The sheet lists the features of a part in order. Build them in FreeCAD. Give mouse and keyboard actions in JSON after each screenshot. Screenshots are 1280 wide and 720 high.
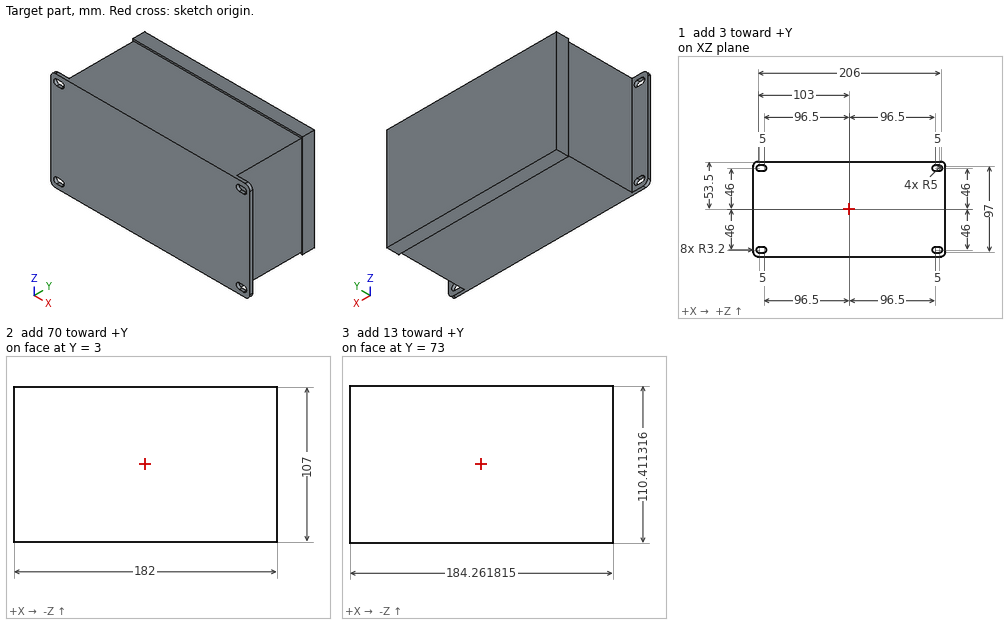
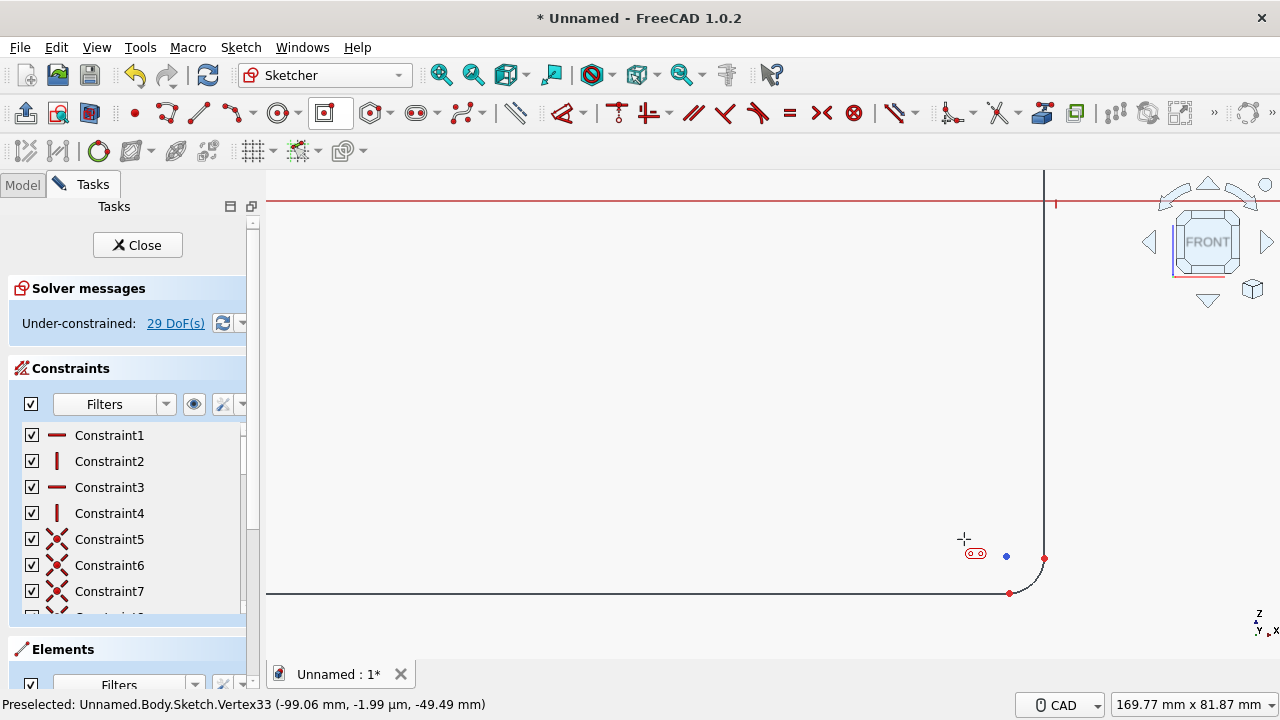
{"action": "left_click", "coordinate": [962, 537]}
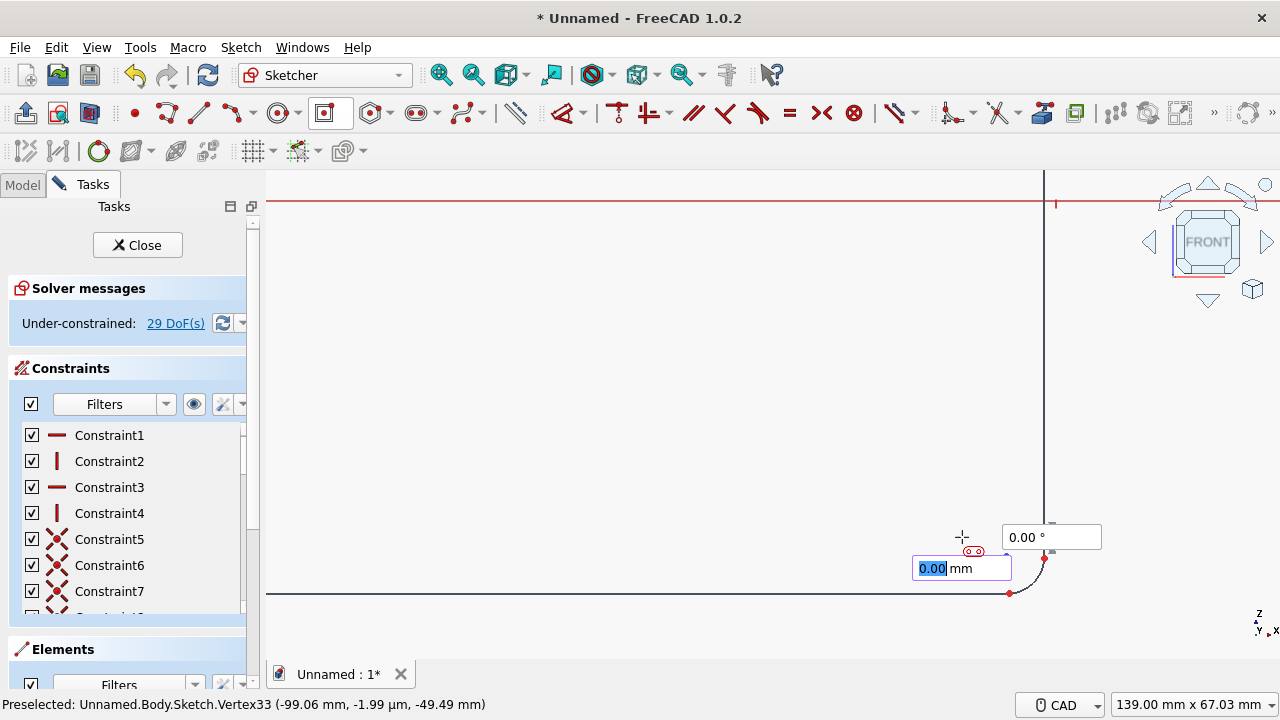
{"action": "left_click", "coordinate": [998, 537]}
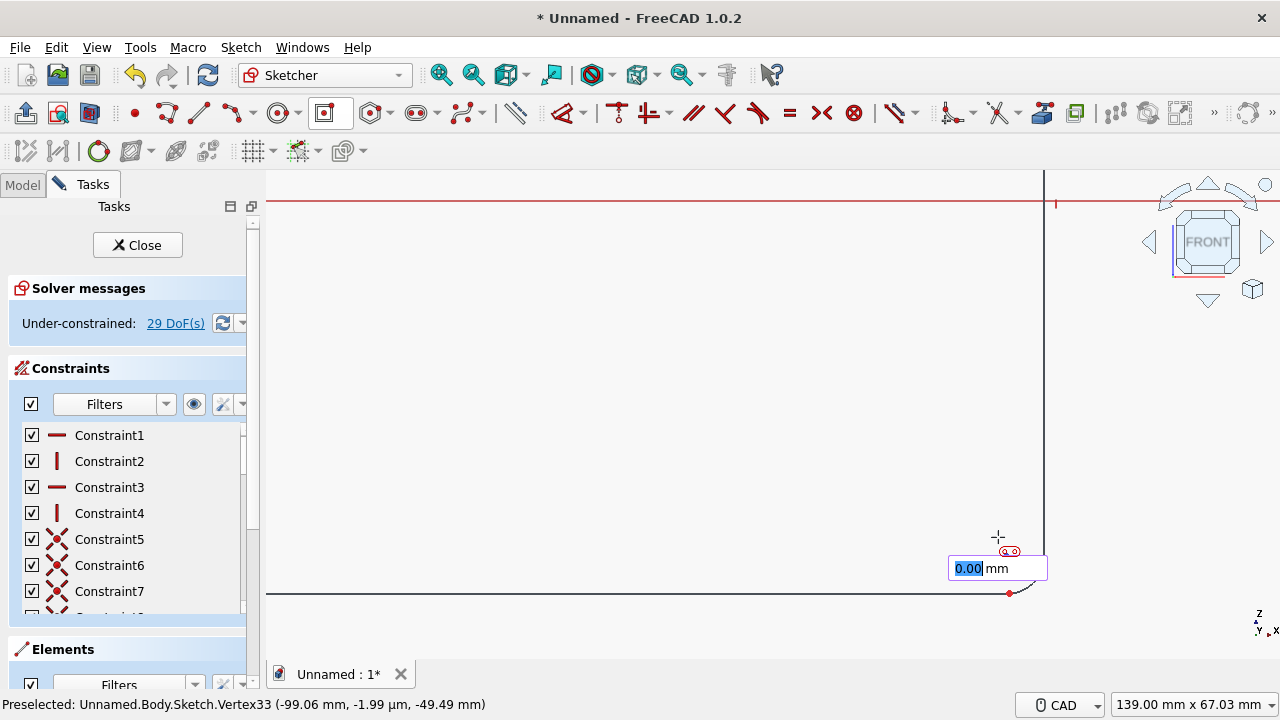
{"action": "left_click", "coordinate": [980, 560]}
{"action": "key", "text": "Escape"}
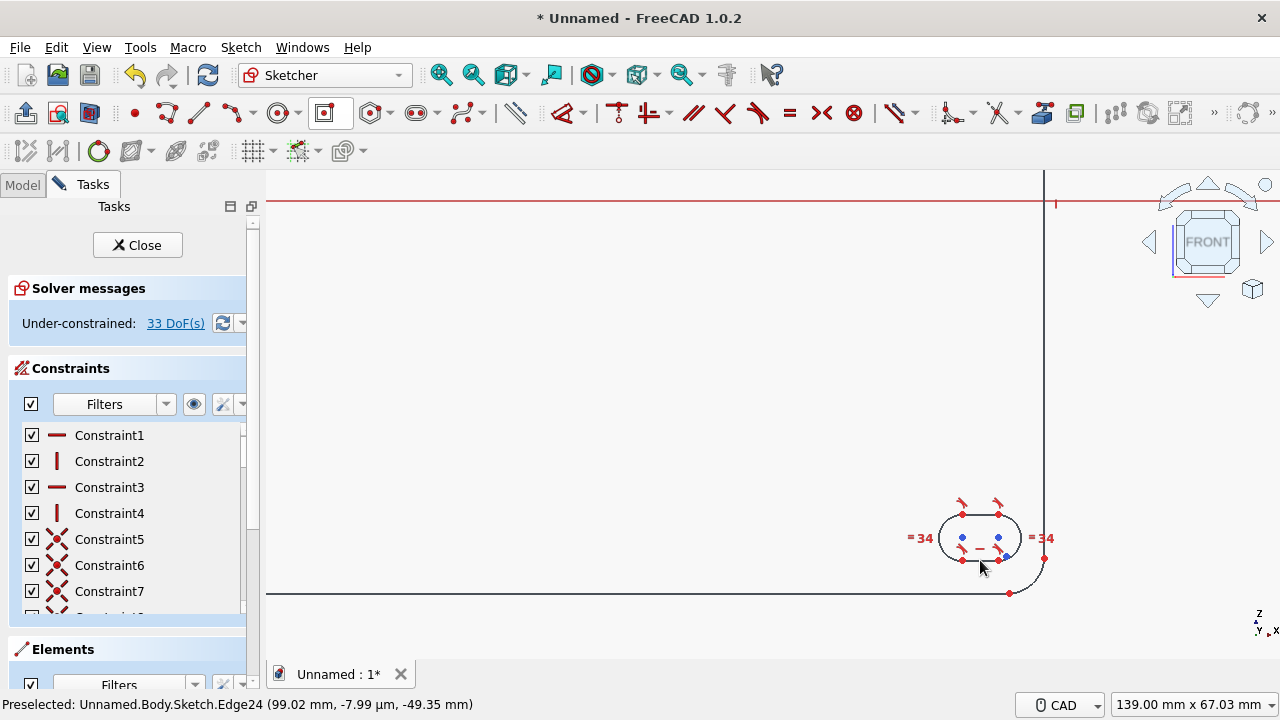
{"action": "scroll", "coordinate": [965, 539], "scroll_direction": "down", "scroll_amount": 5}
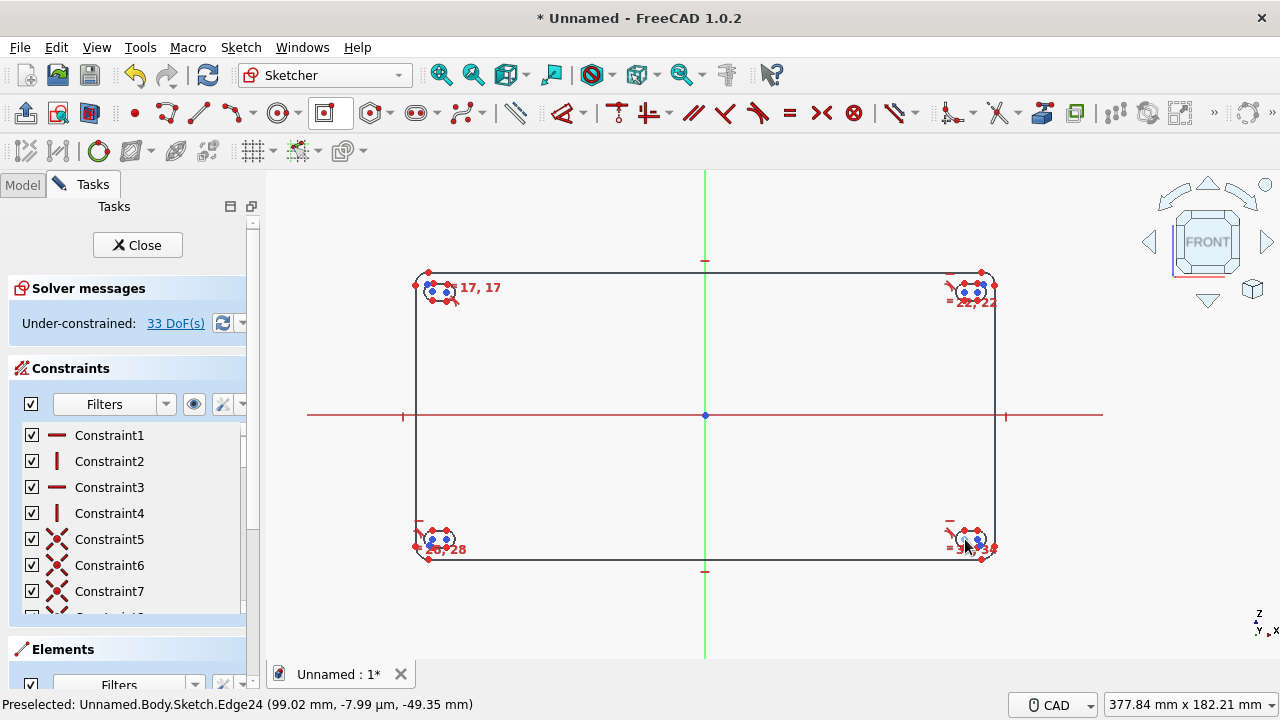
{"action": "left_click", "coordinate": [595, 273]}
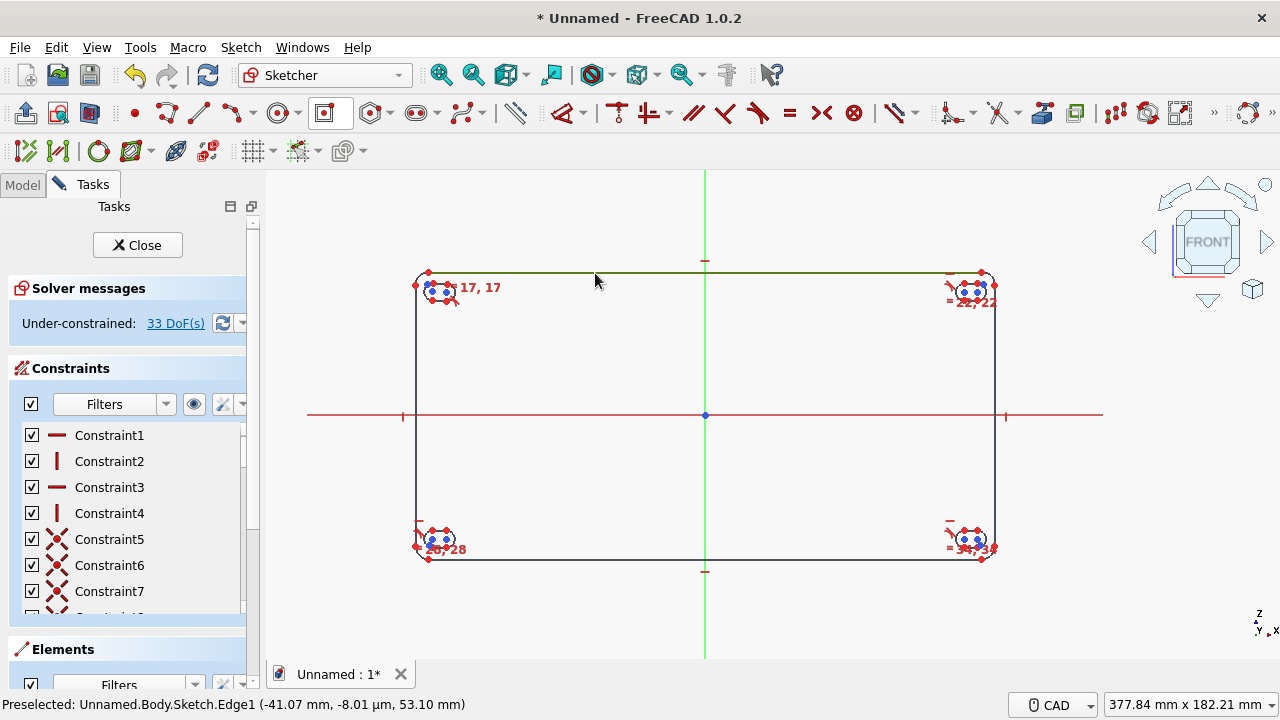
{"action": "scroll", "coordinate": [991, 276], "scroll_direction": "up", "scroll_amount": 2}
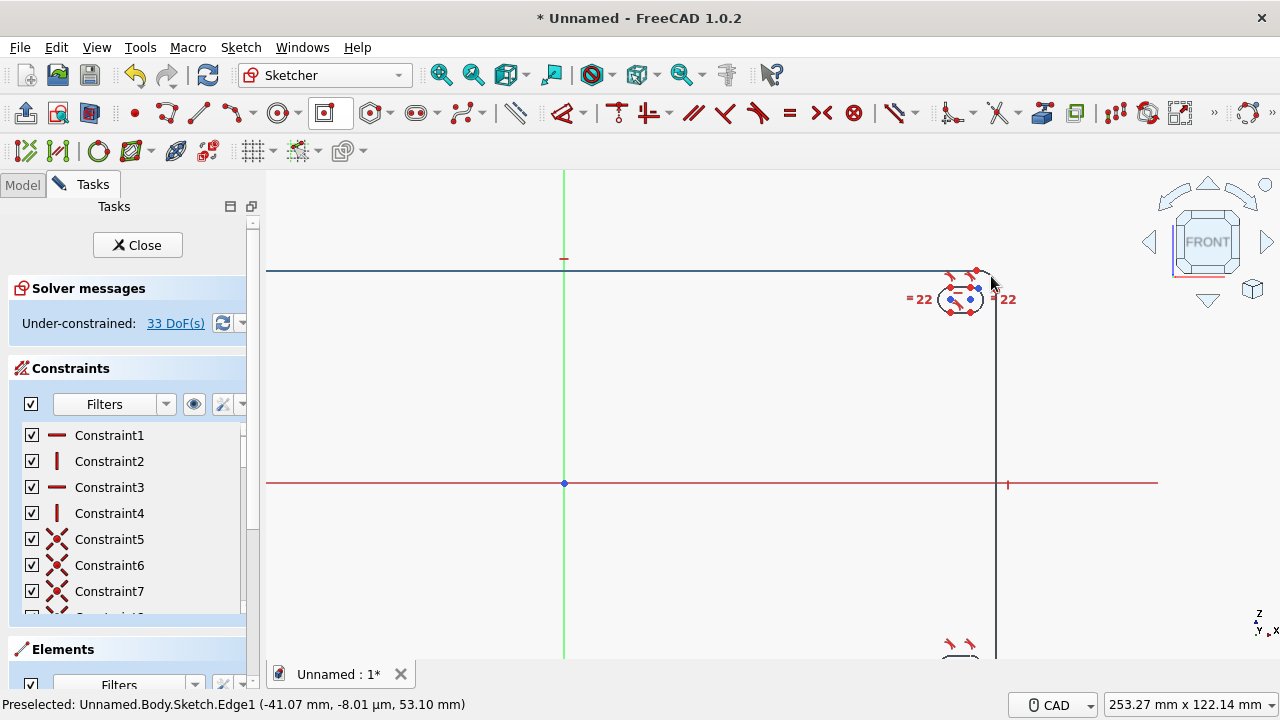
{"action": "left_click", "coordinate": [991, 276]}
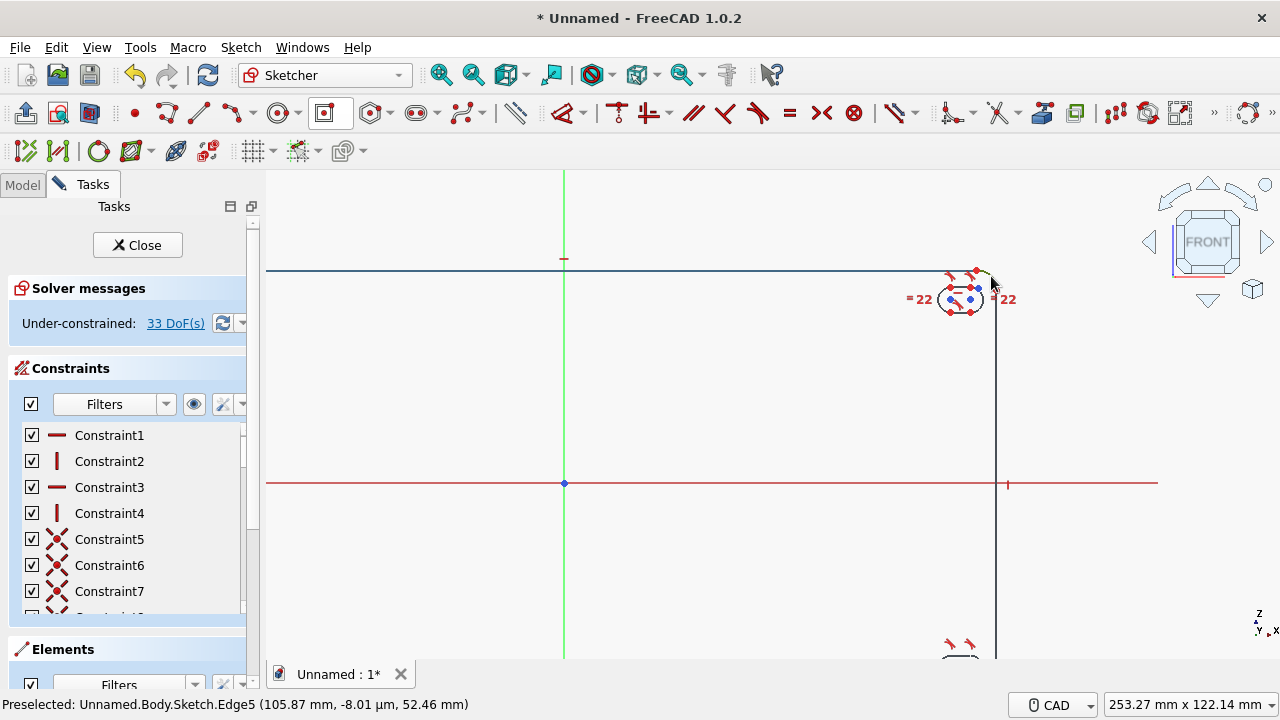
{"action": "left_click", "coordinate": [758, 114]}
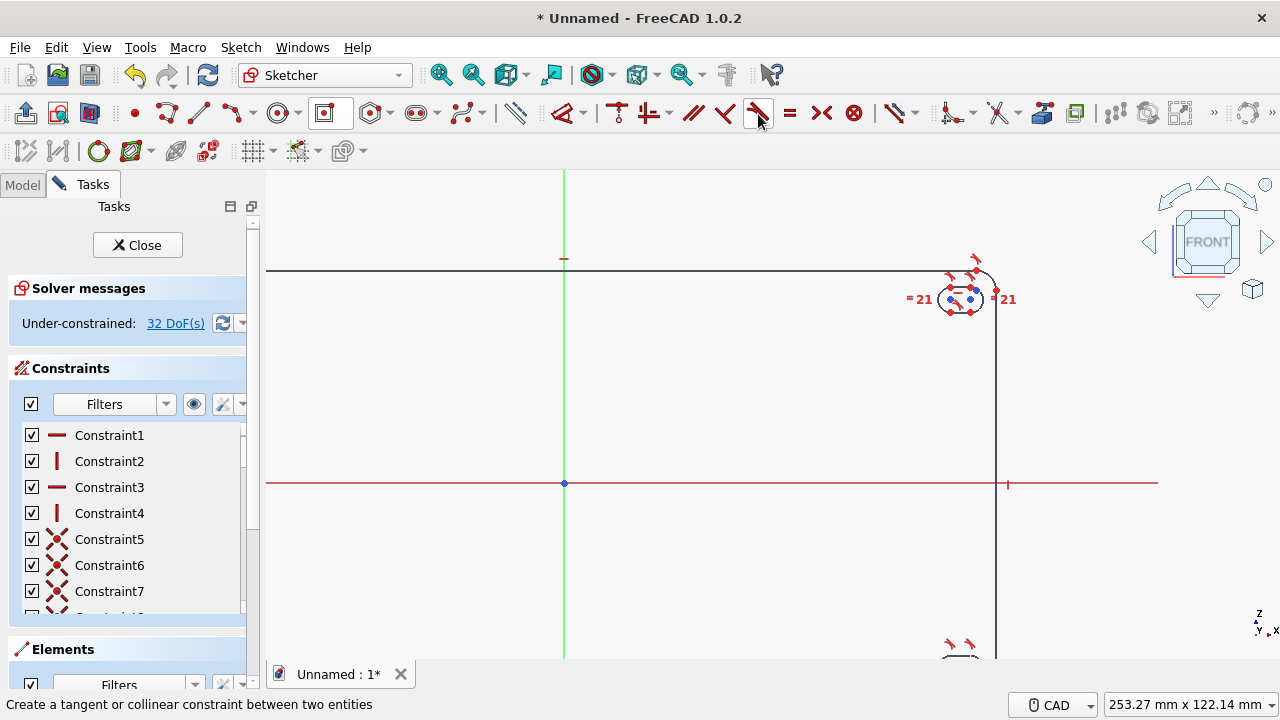
{"action": "left_click", "coordinate": [399, 271]}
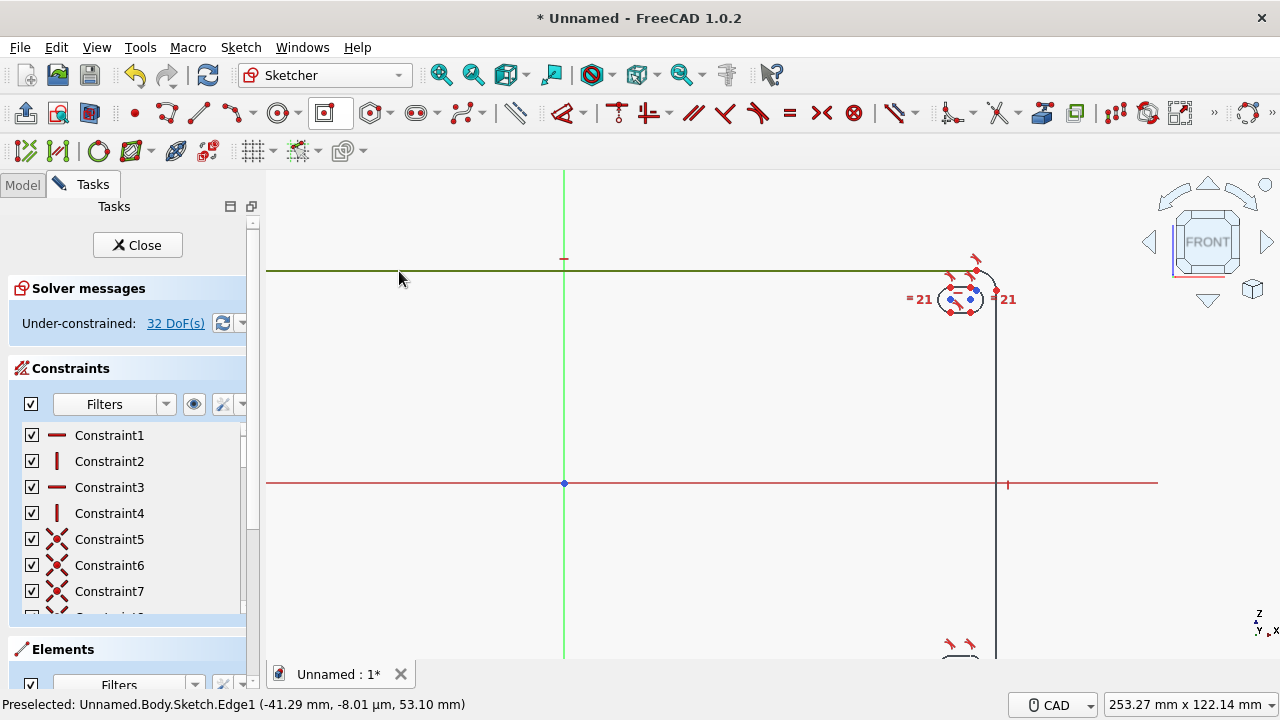
{"action": "scroll", "coordinate": [990, 274], "scroll_direction": "down", "scroll_amount": 2}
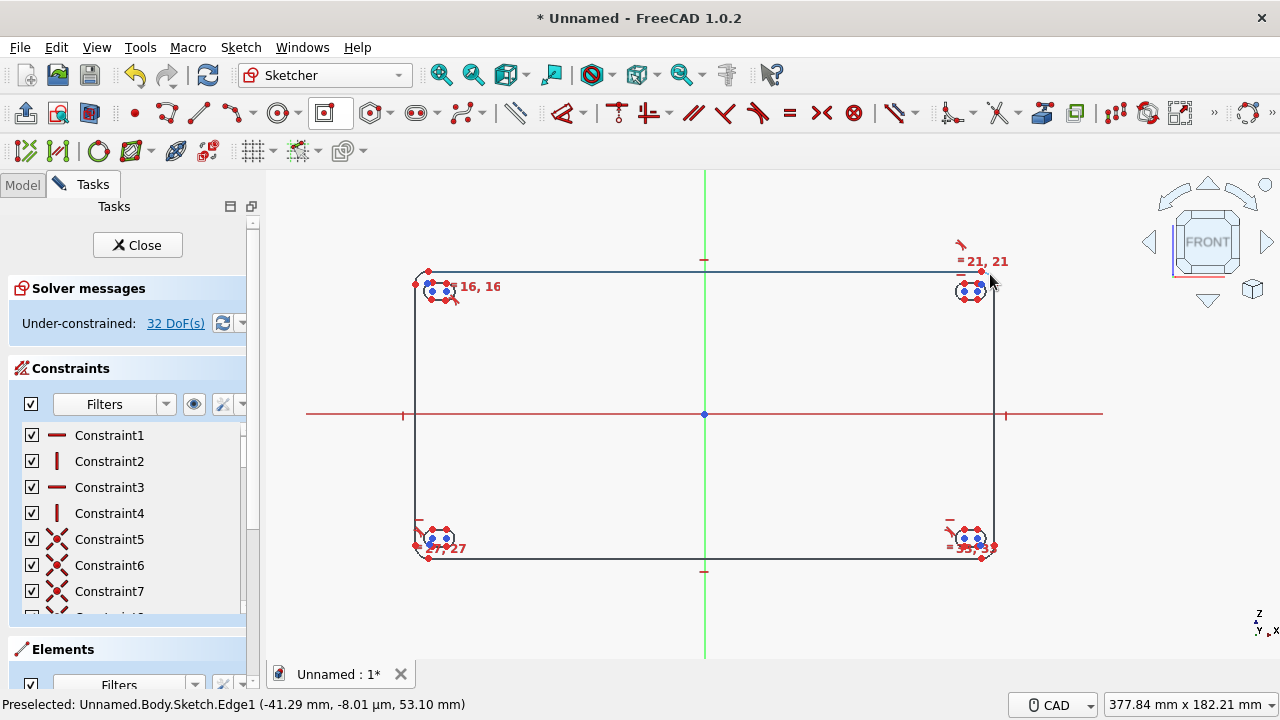
{"action": "scroll", "coordinate": [422, 273], "scroll_direction": "up", "scroll_amount": 4}